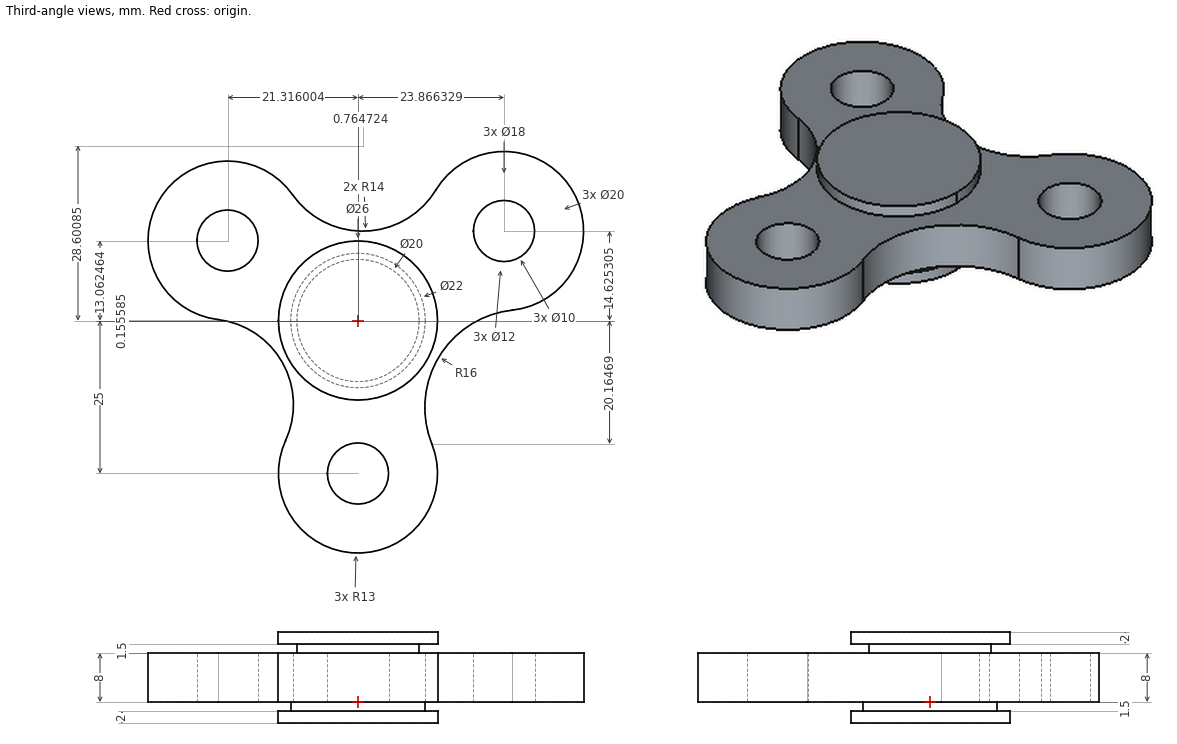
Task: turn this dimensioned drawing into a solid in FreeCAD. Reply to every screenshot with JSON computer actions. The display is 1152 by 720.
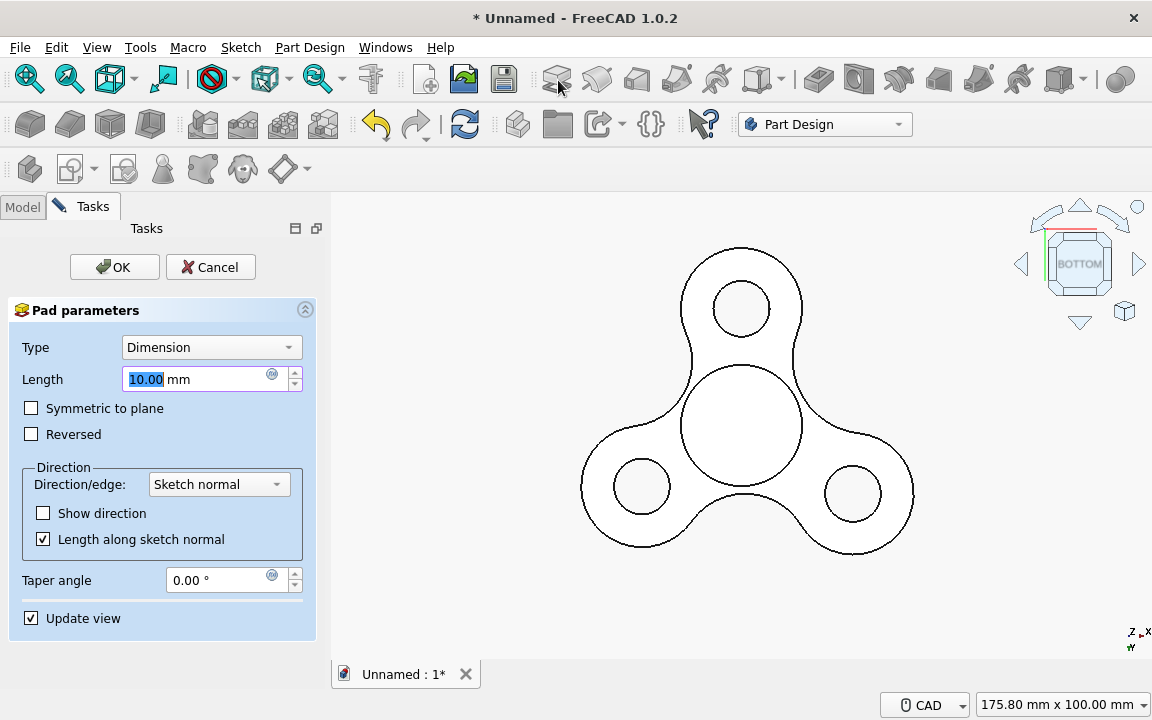
{"action": "type", "text": "8"}
{"action": "key", "text": "Tab"}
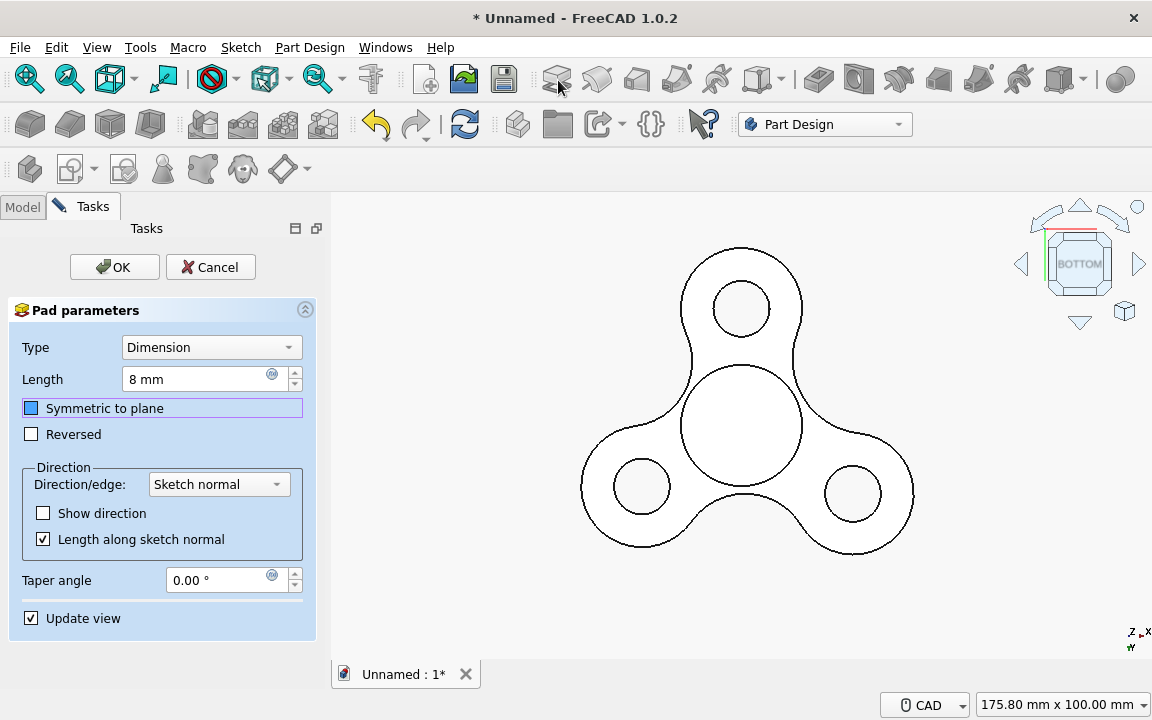
{"action": "left_click", "coordinate": [30, 434]}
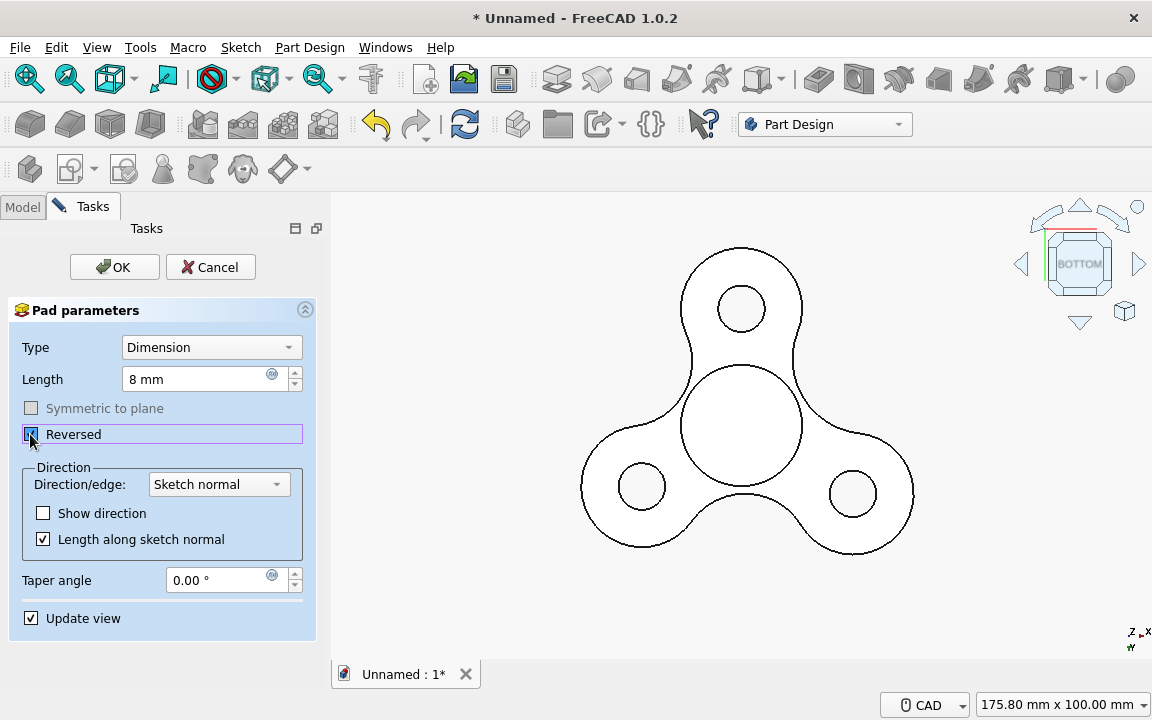
{"action": "left_click", "coordinate": [115, 267]}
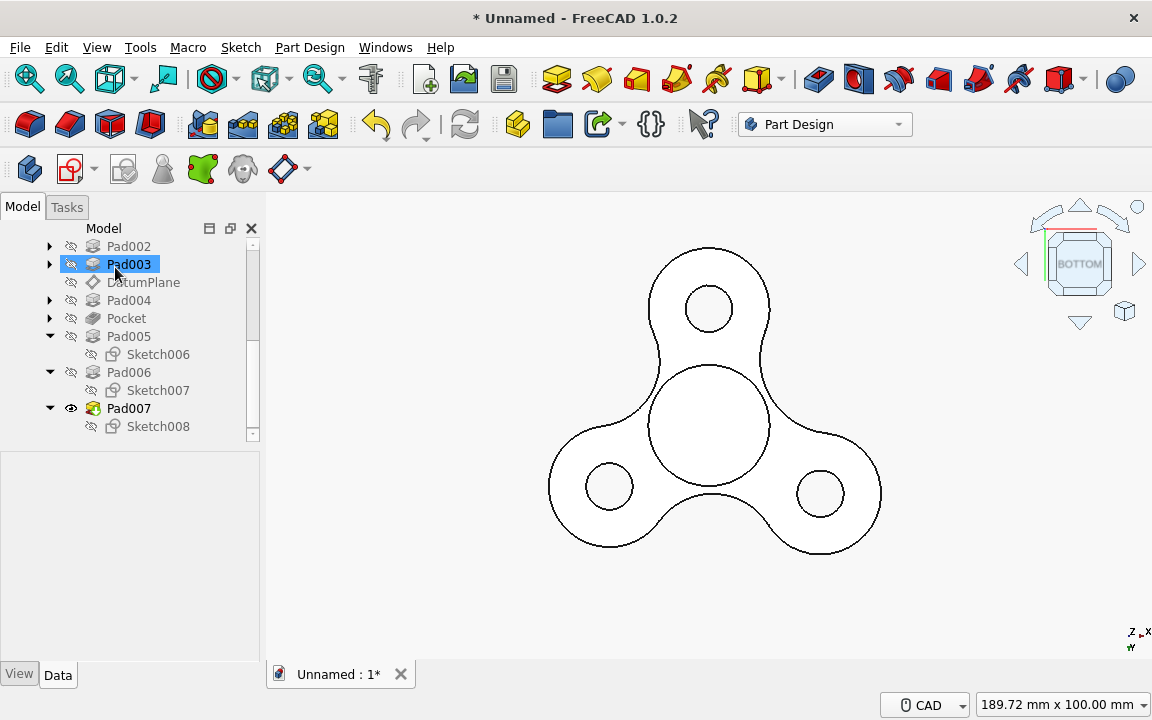
{"action": "key", "text": "0"}